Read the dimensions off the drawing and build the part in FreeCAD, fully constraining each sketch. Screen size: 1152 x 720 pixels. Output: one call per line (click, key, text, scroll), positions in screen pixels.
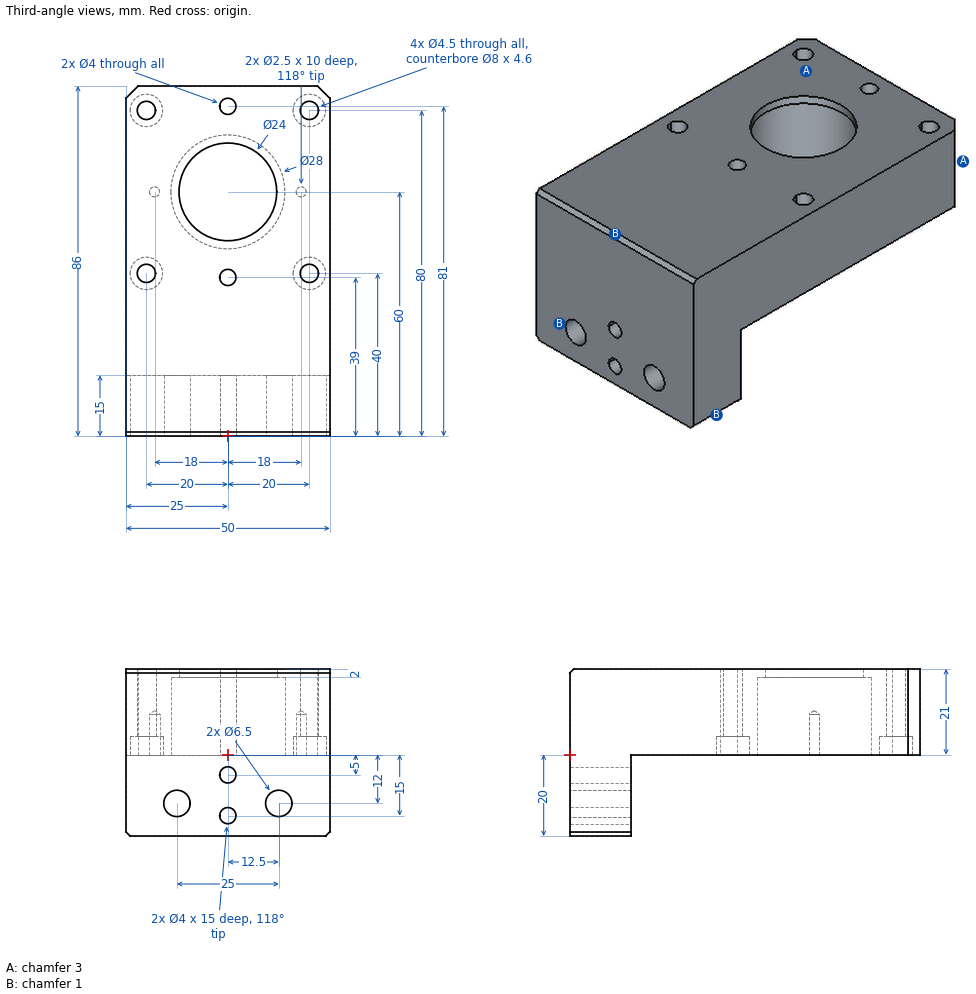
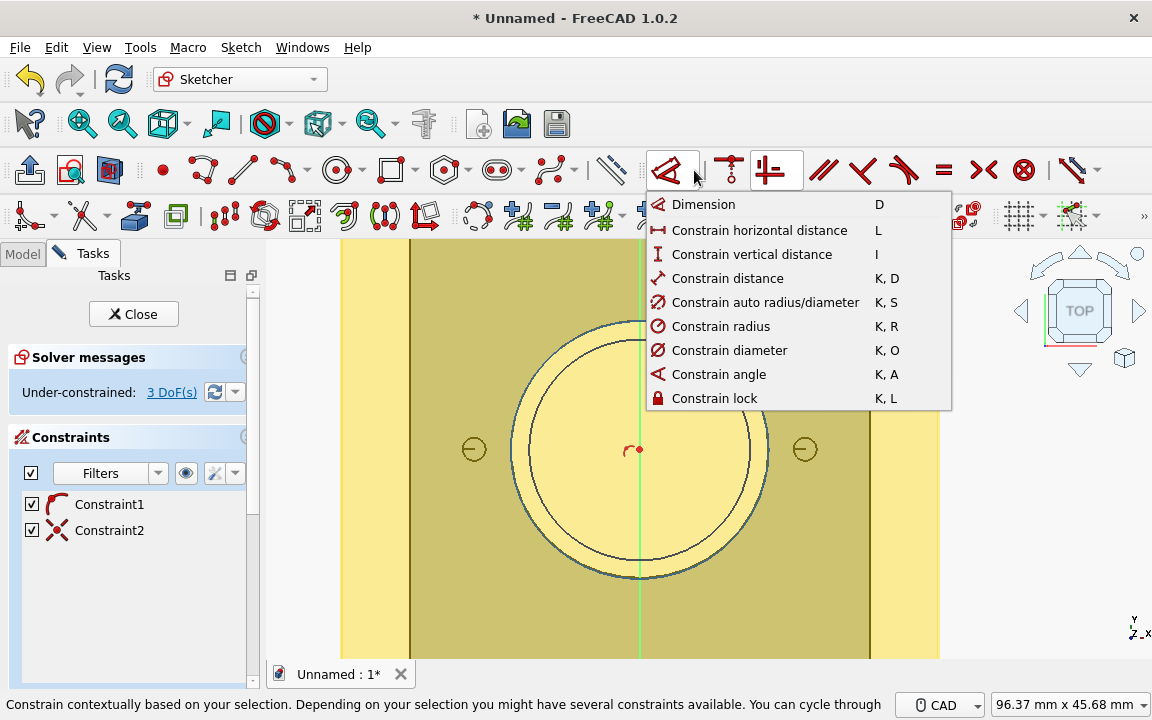
click(799, 350)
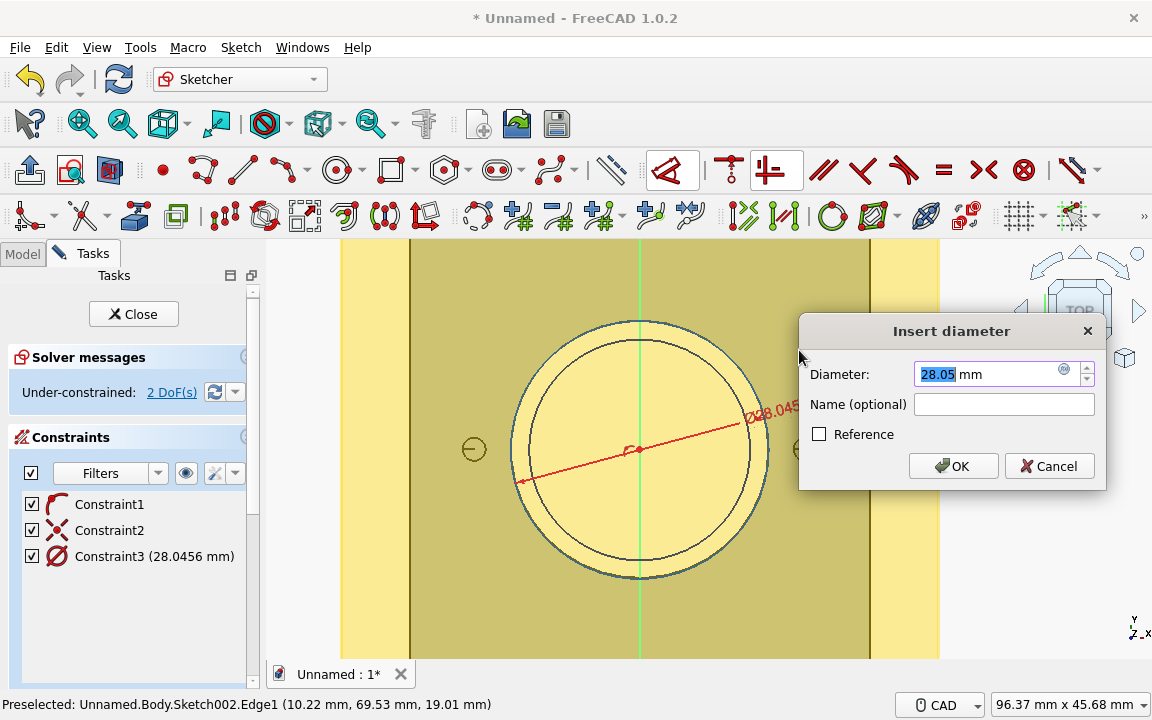
text(28)
key(Return)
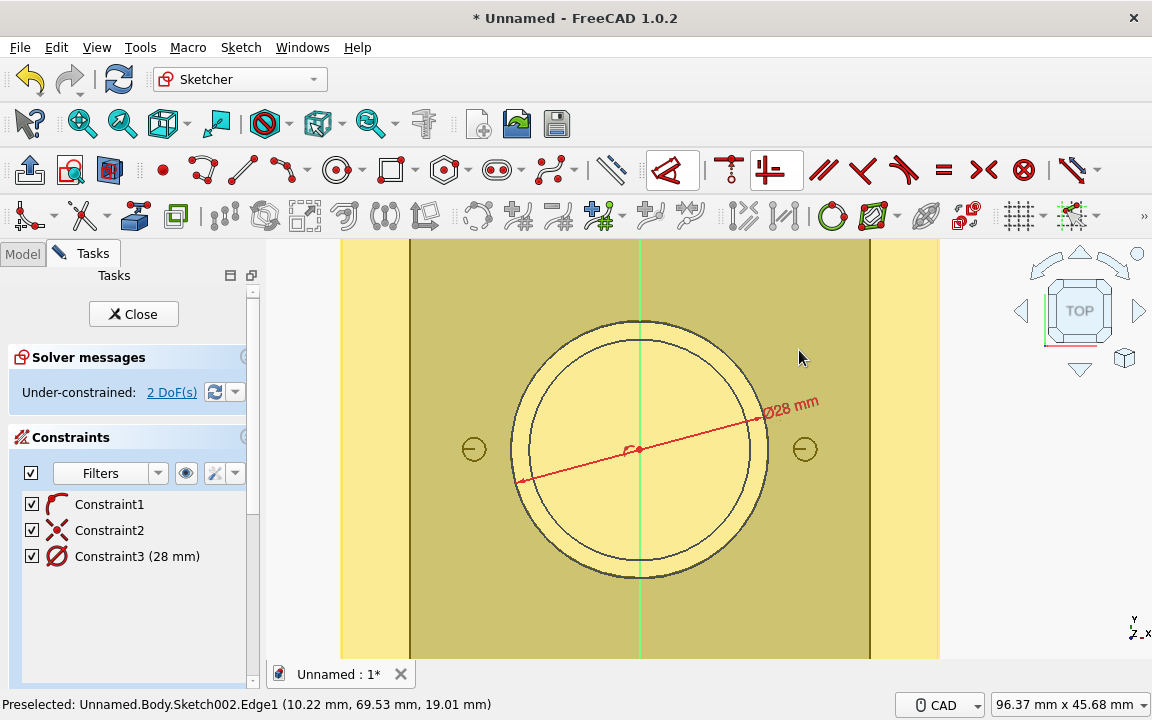
click(718, 372)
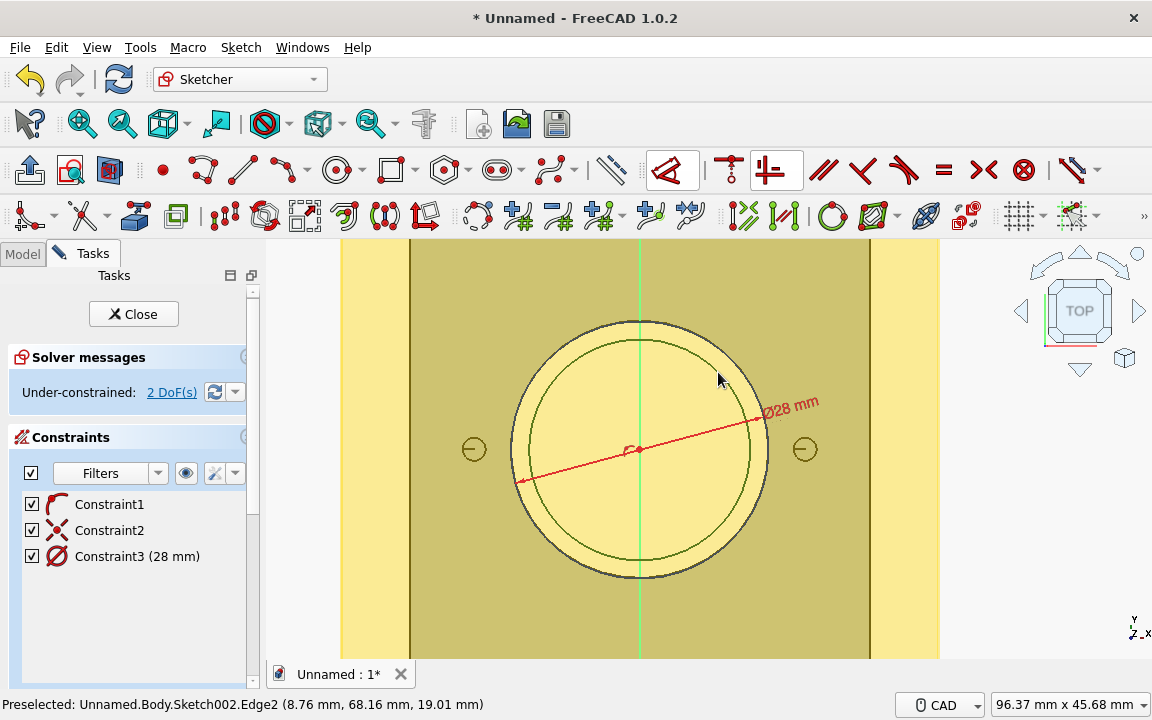
key(k)
key(o)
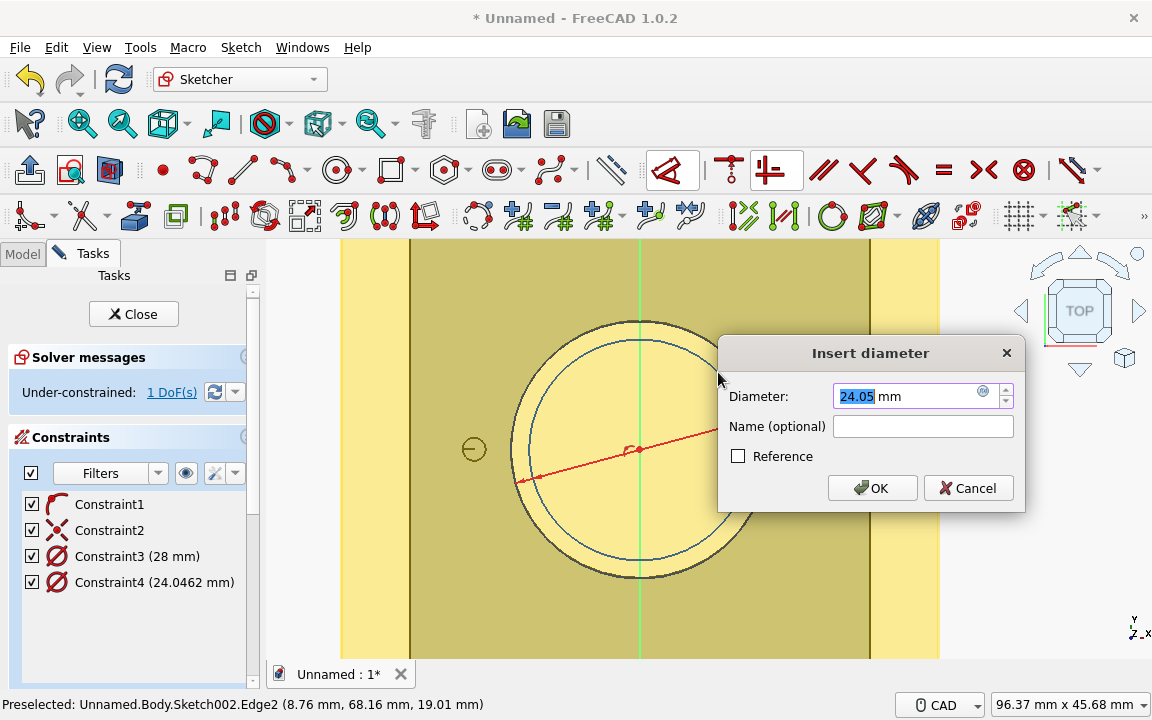
text(24)
key(Return)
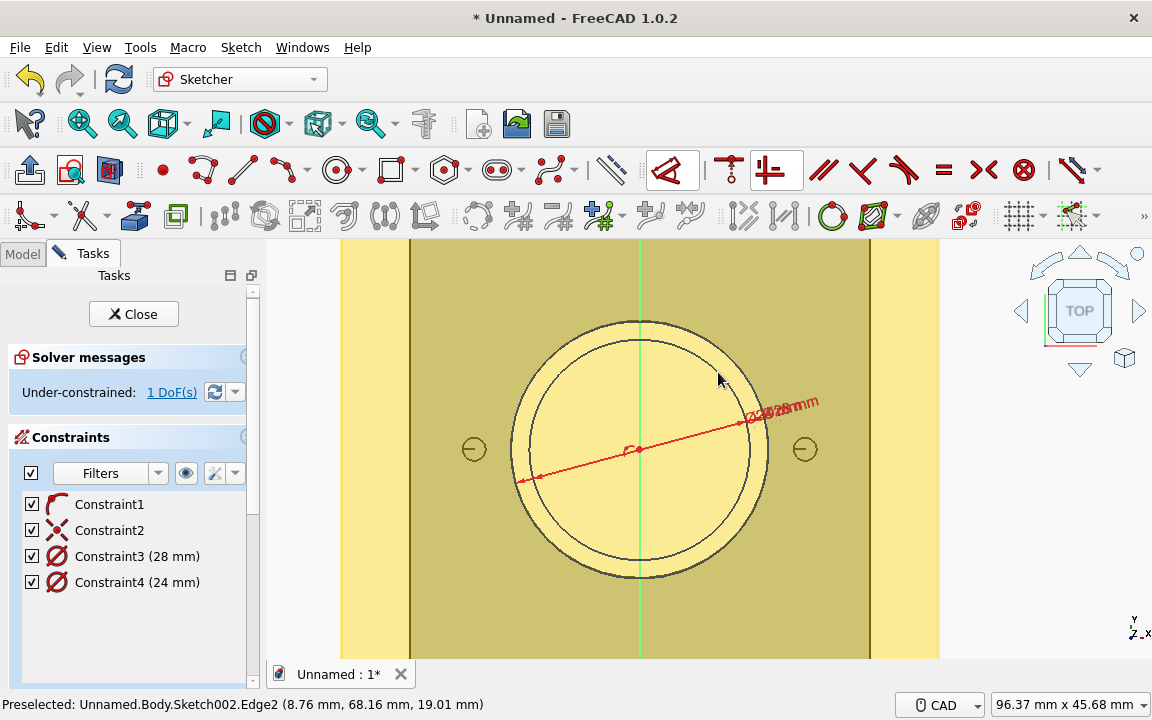
click(640, 450)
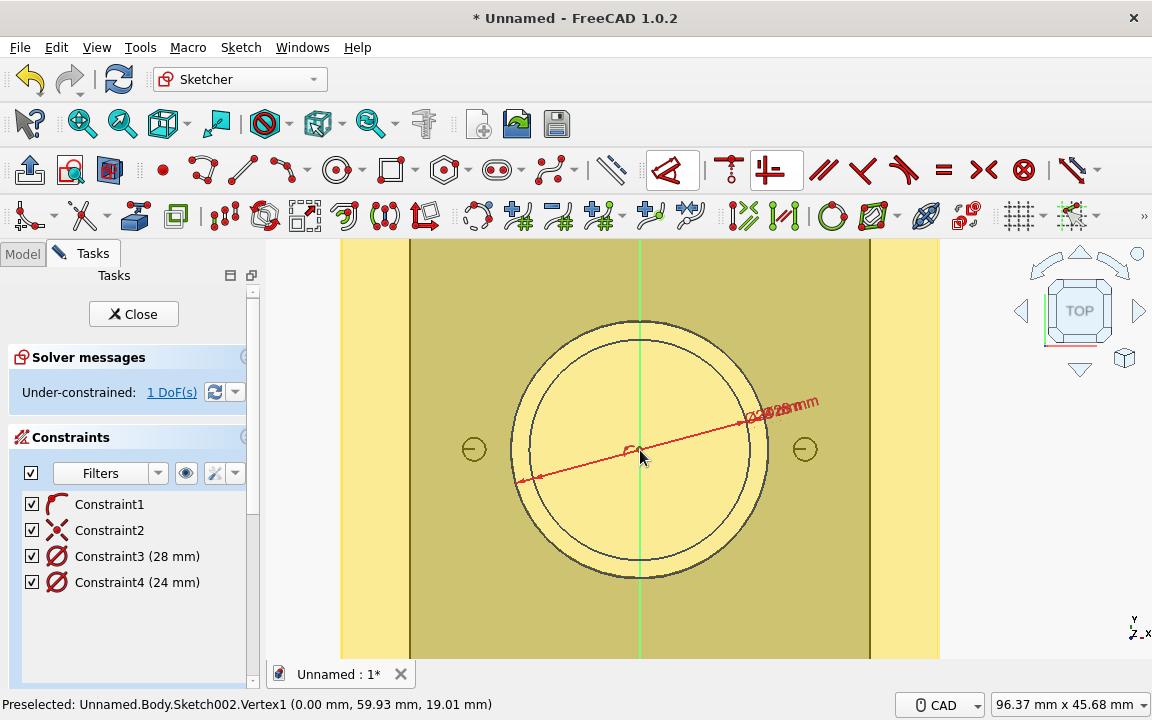
click(694, 170)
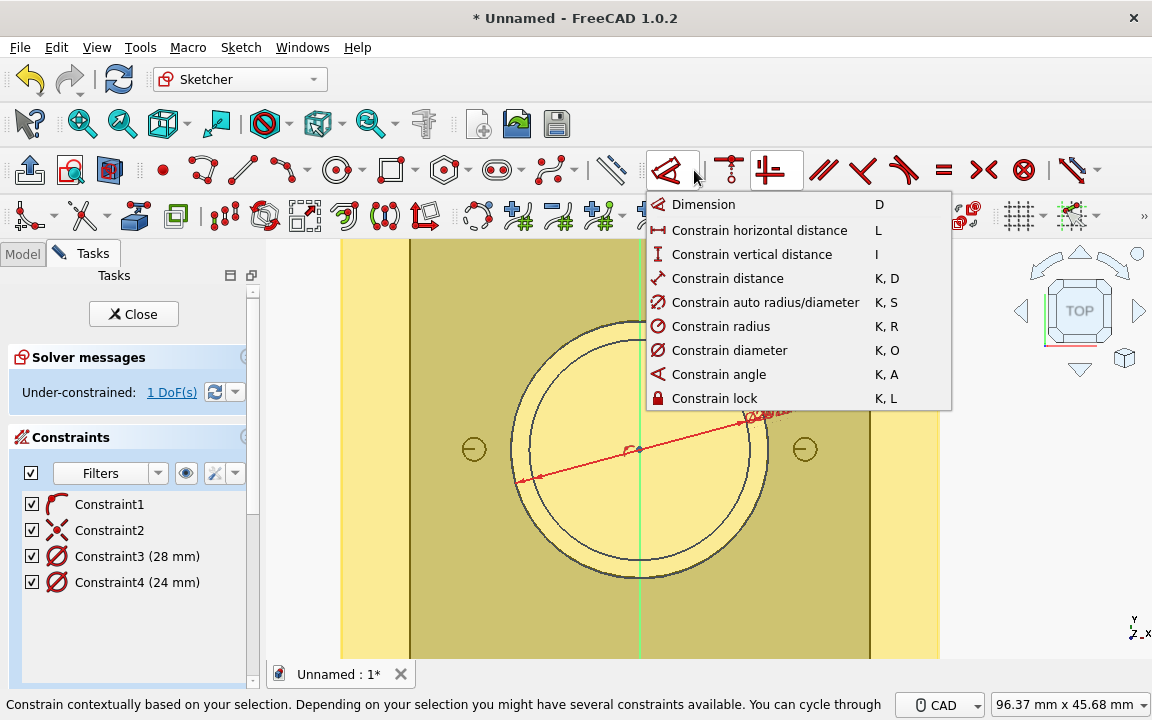
click(799, 254)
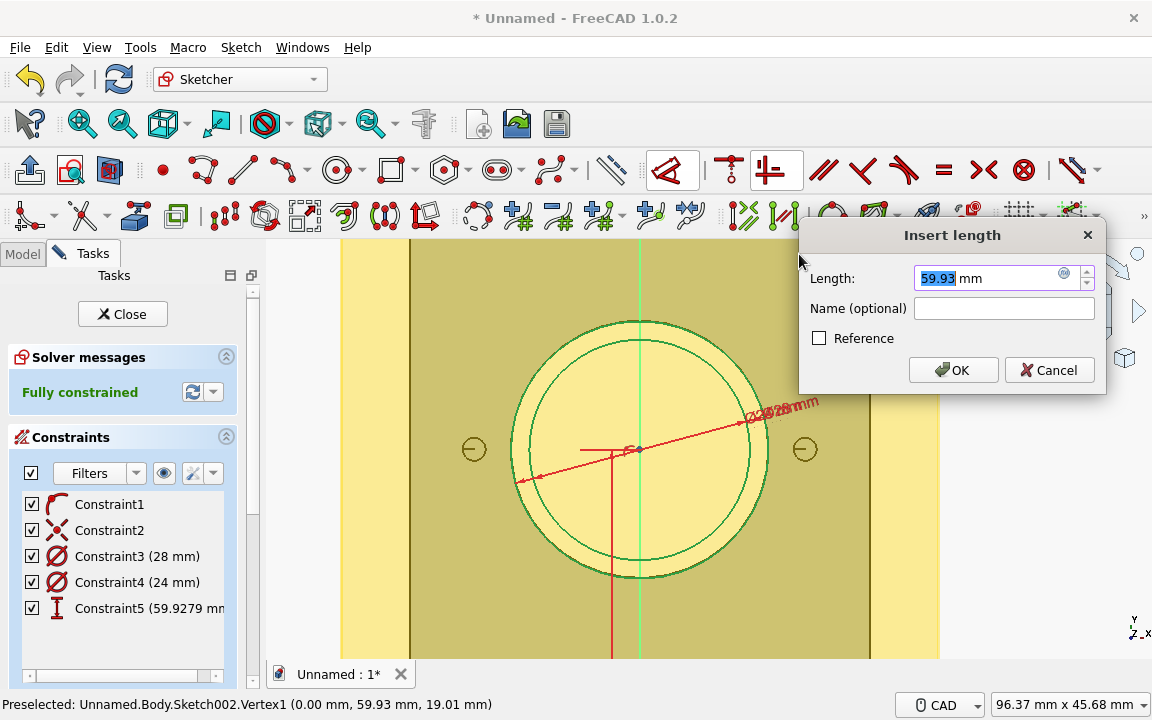
text(60)
key(Return)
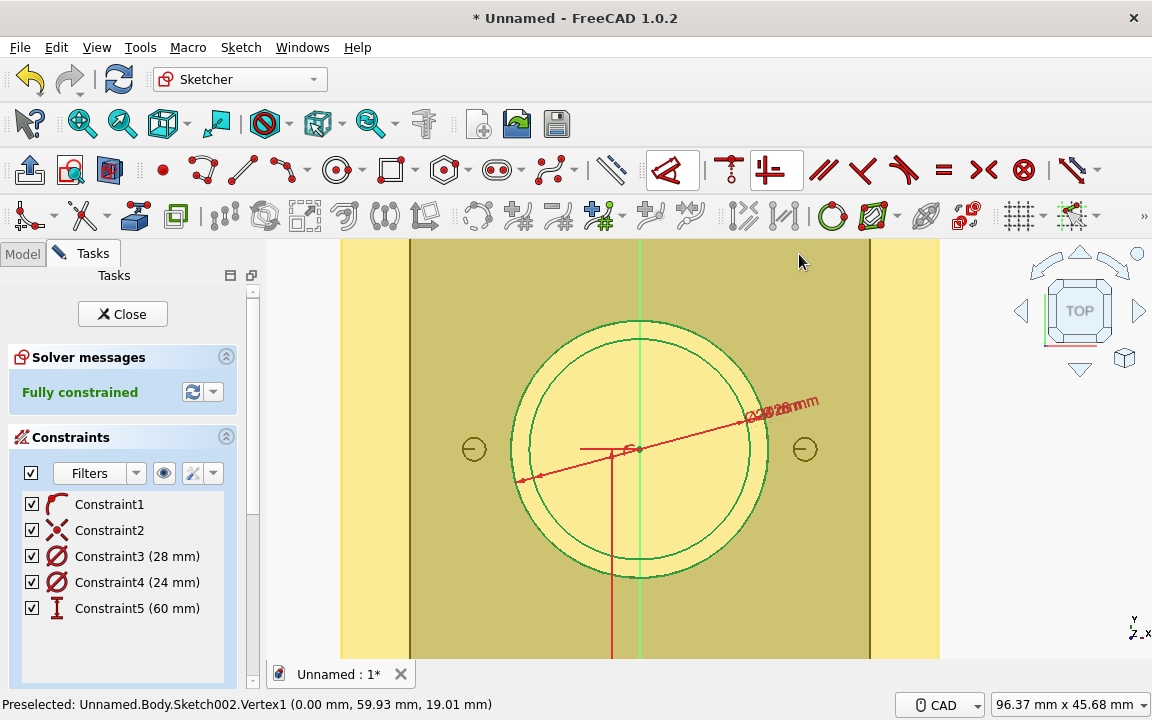
click(123, 314)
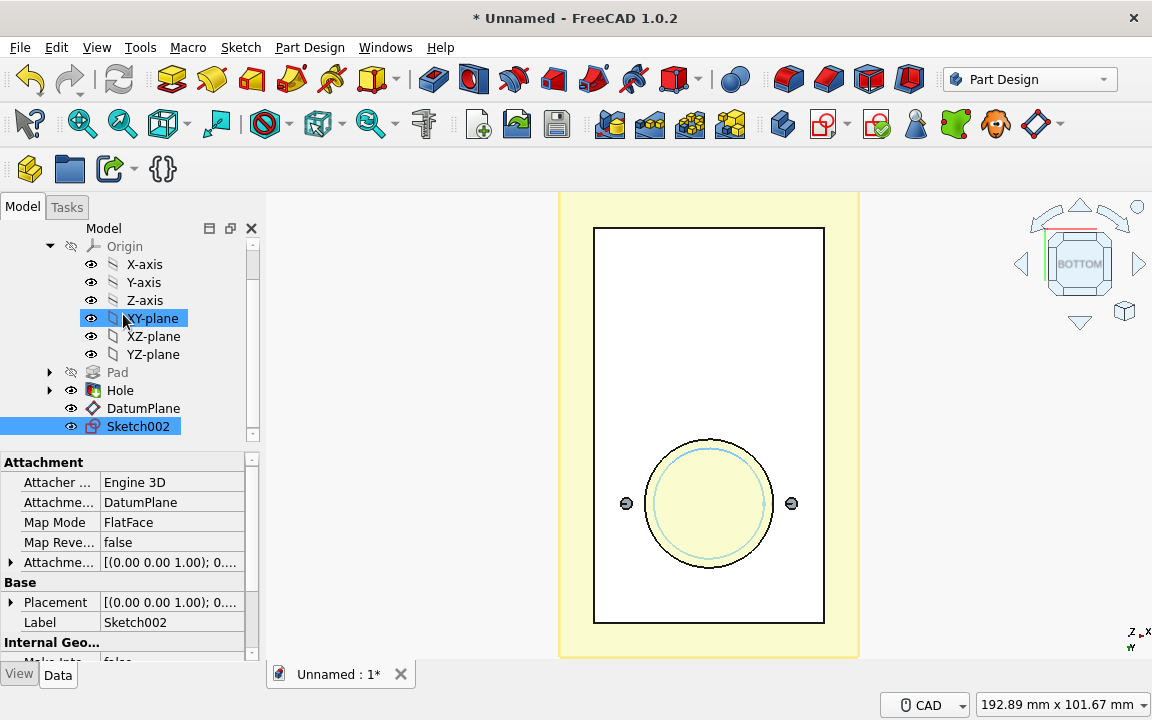
click(172, 80)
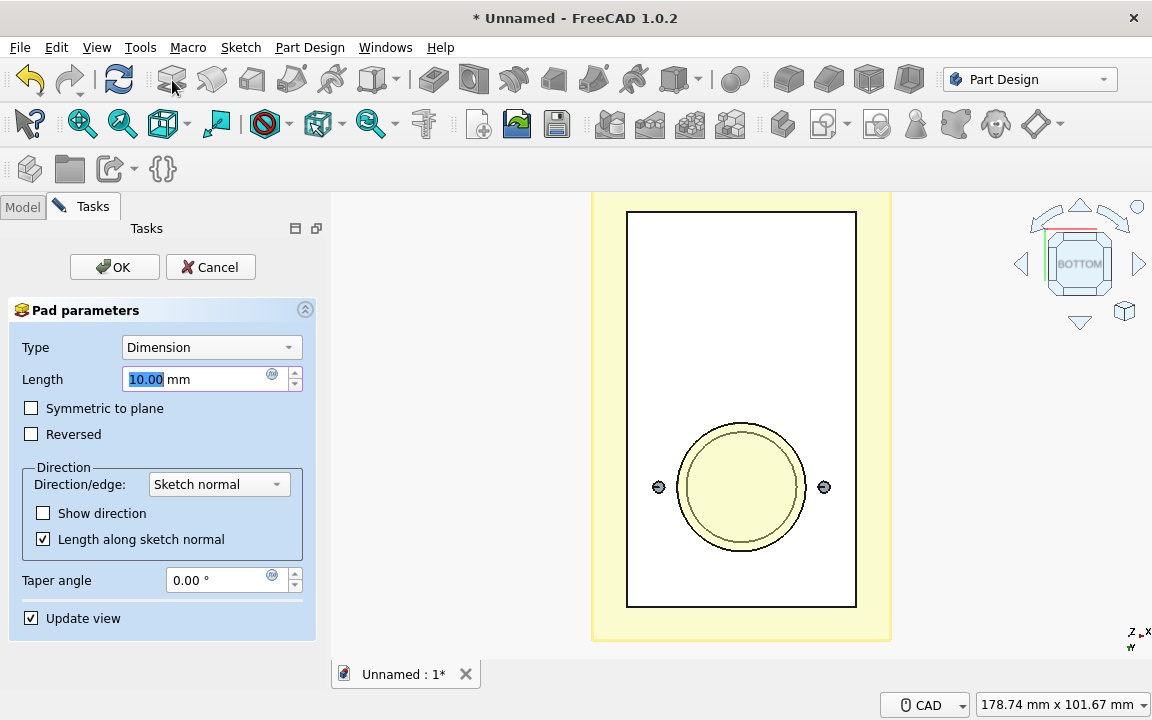
text(2)
key(Tab)